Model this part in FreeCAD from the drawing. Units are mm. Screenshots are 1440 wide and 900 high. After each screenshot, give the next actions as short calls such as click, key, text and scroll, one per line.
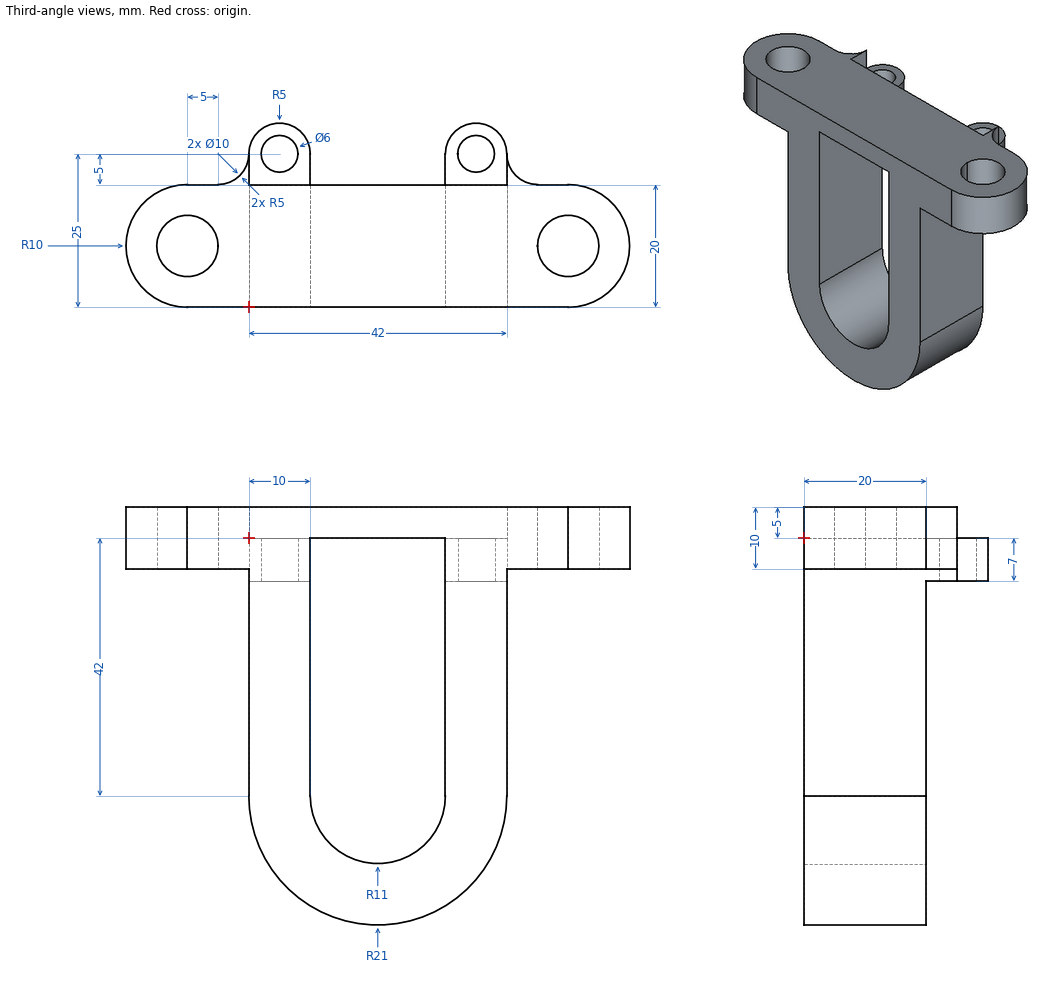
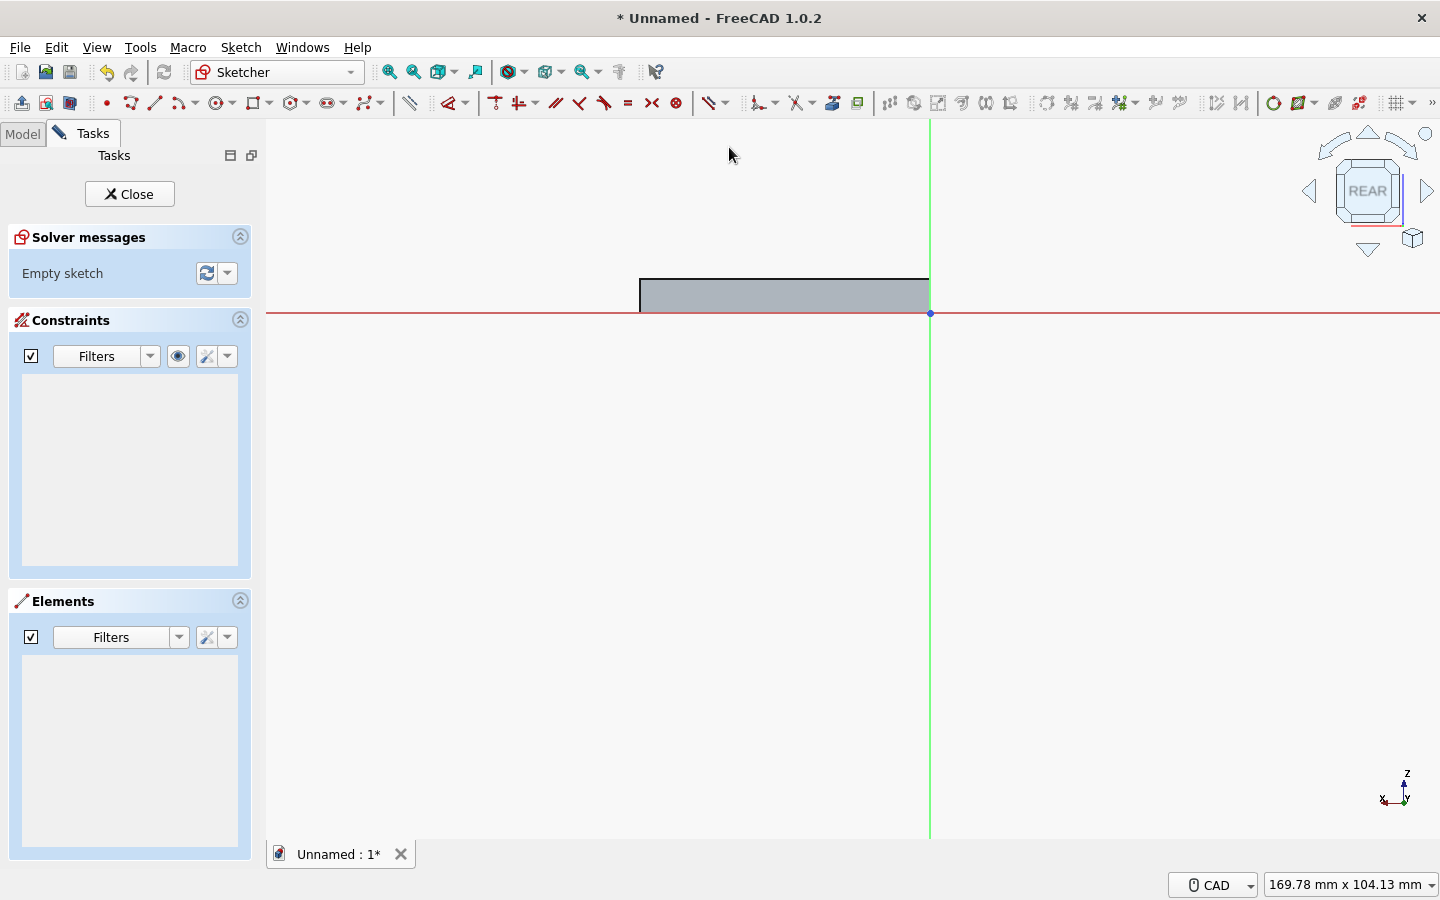
click(132, 104)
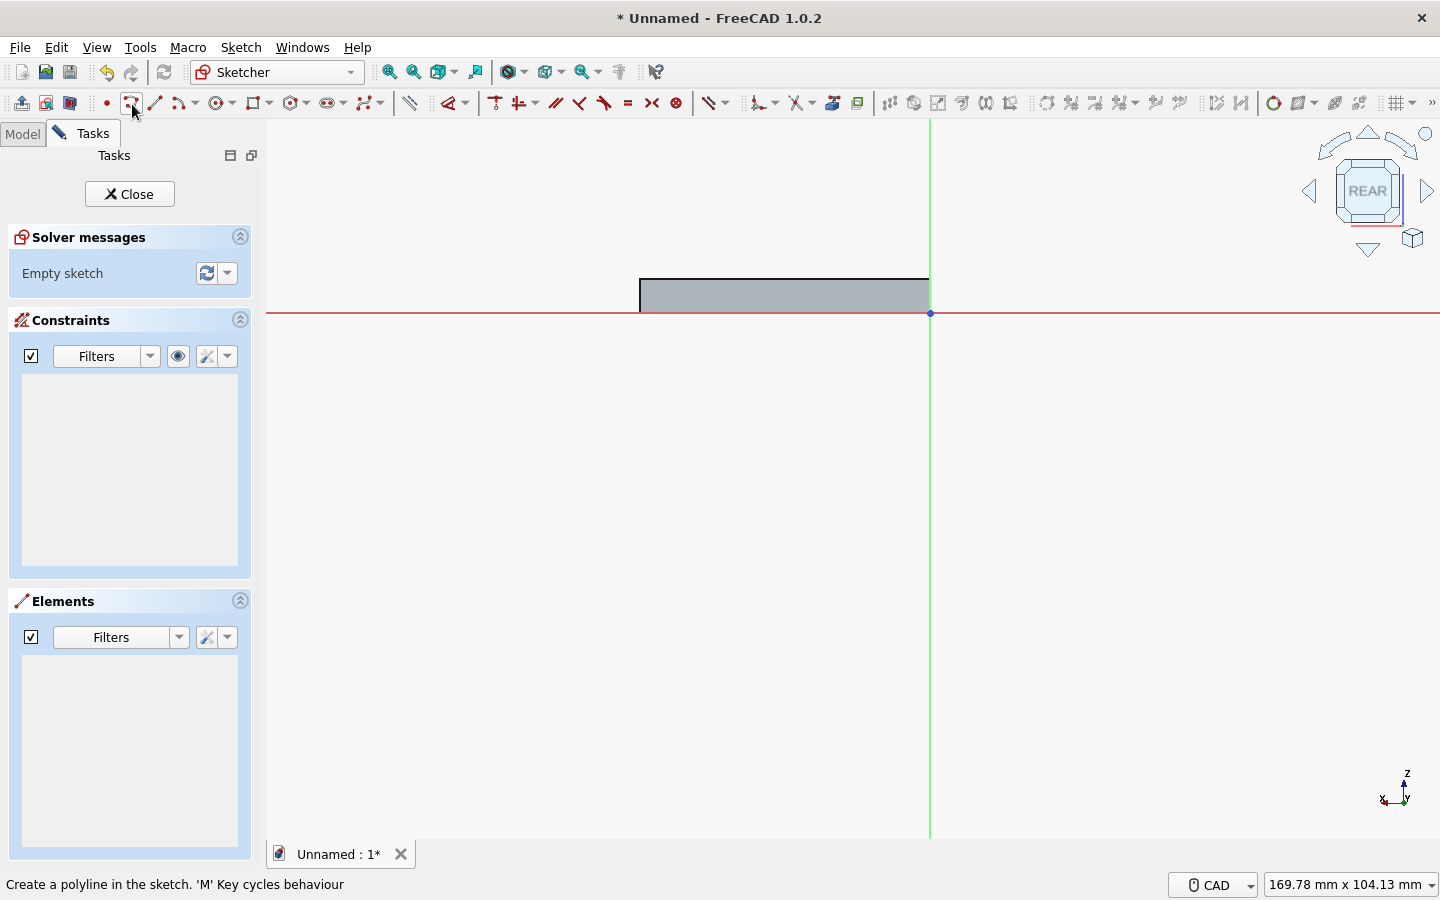
click(930, 604)
click(930, 313)
click(640, 322)
click(640, 604)
right_click(640, 604)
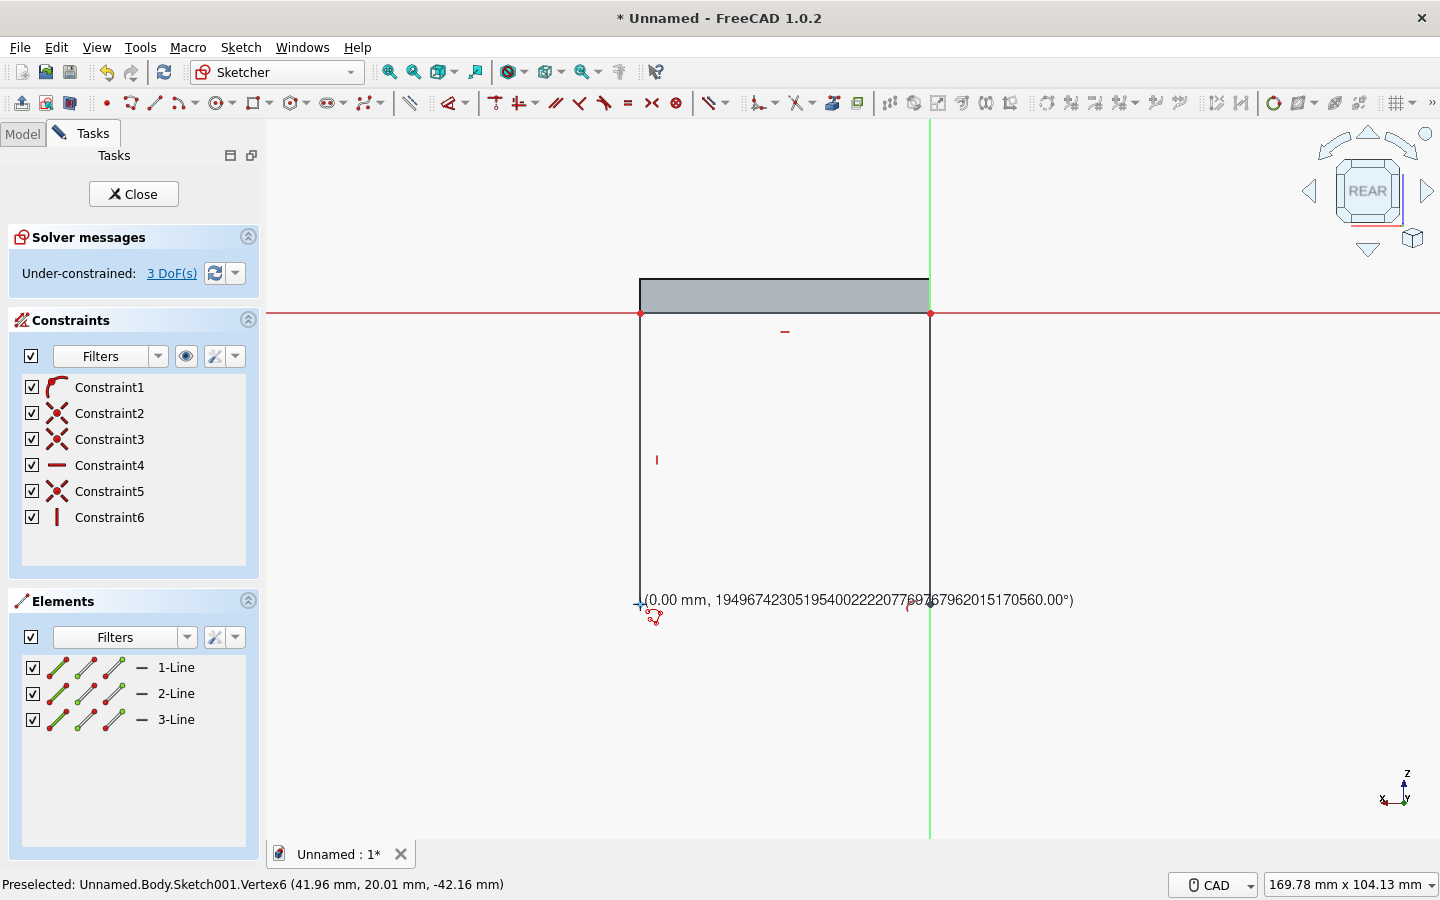
click(198, 104)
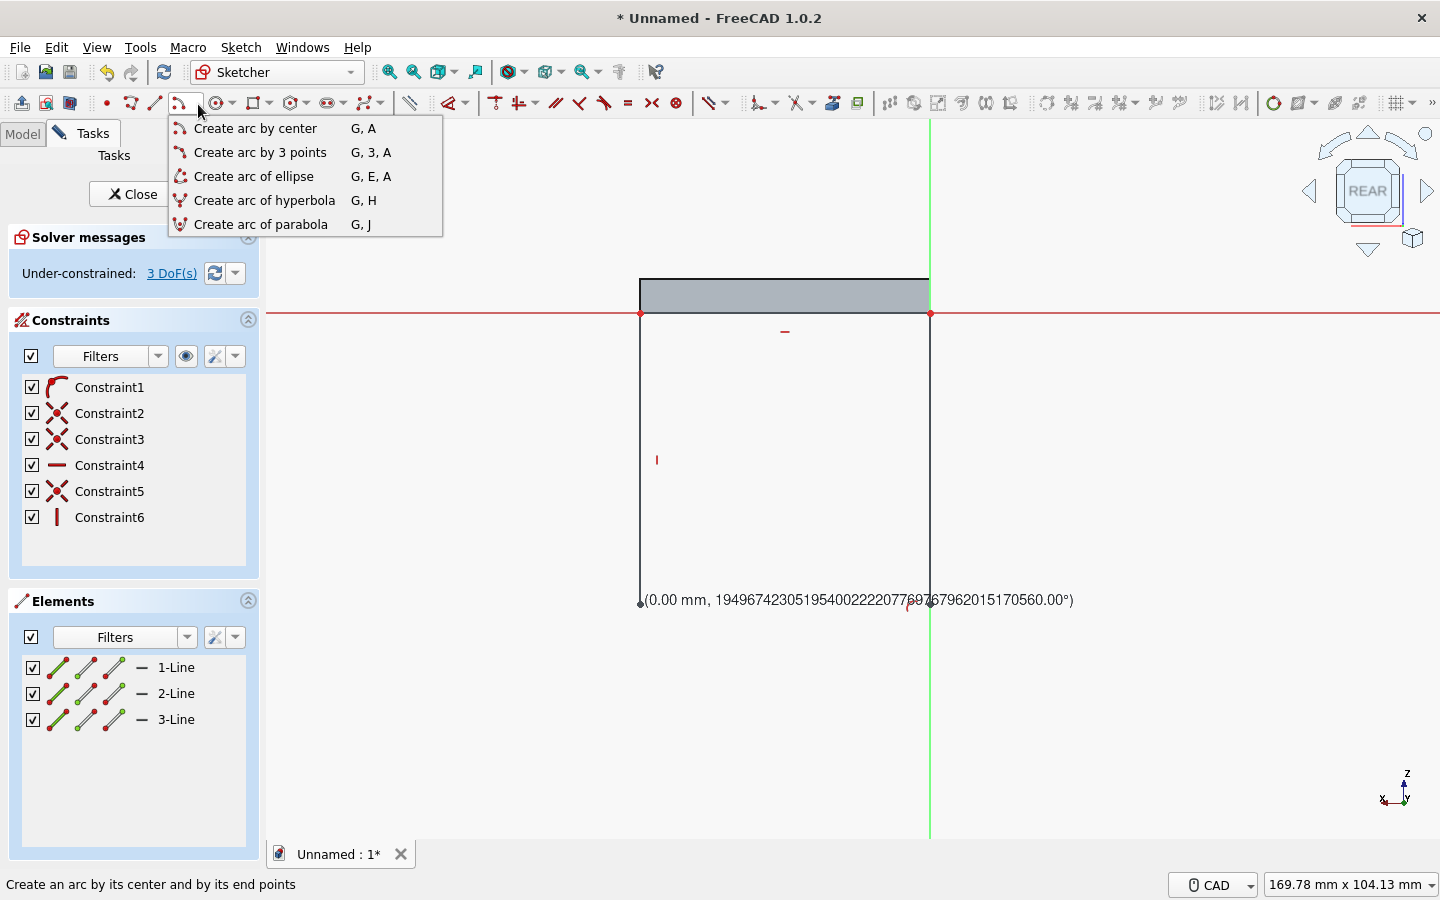
click(306, 152)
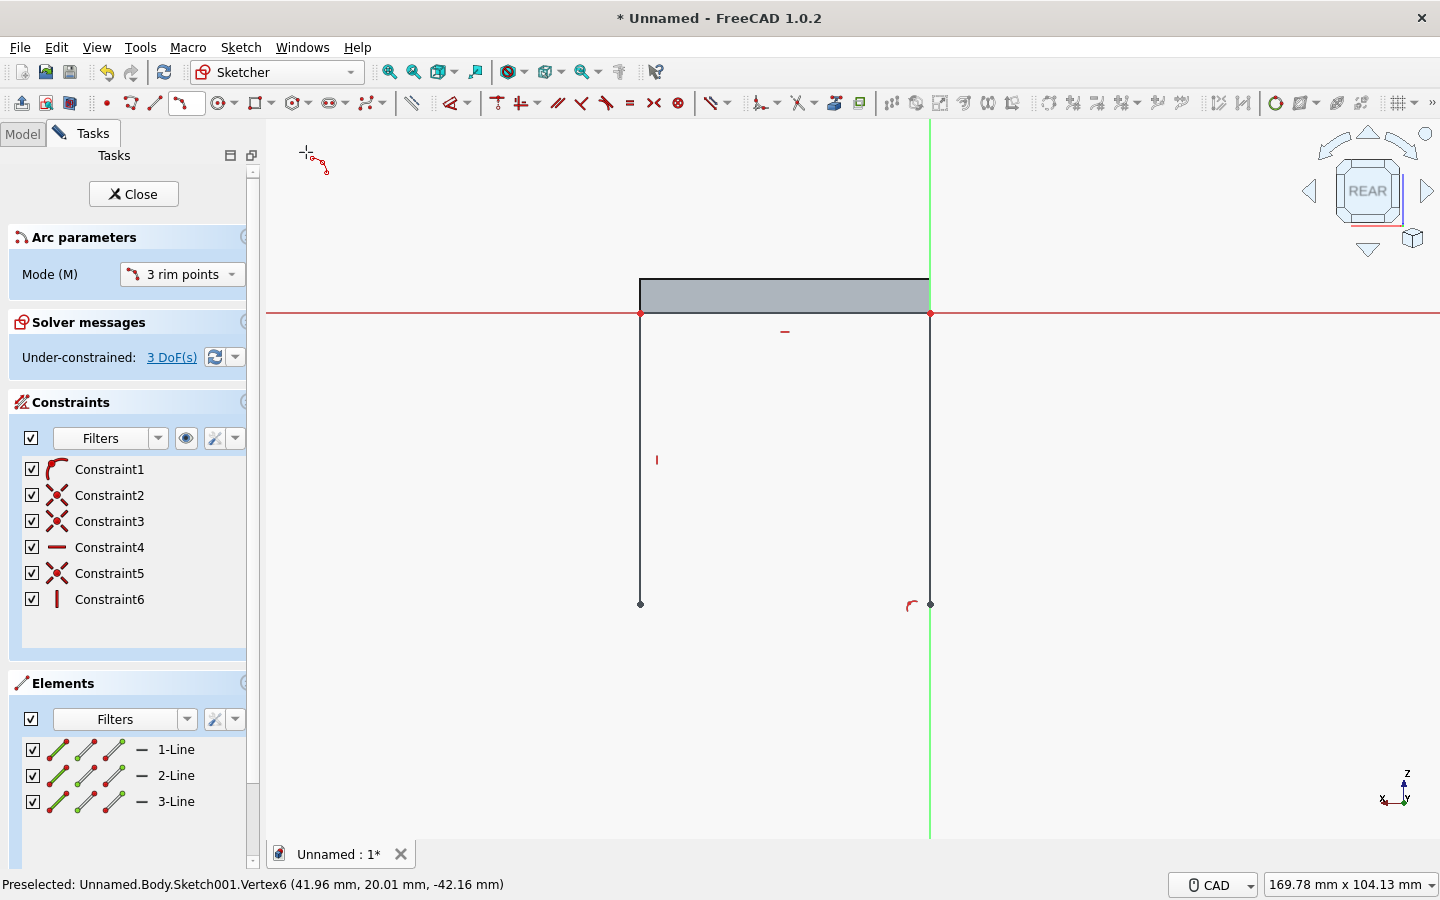
click(640, 605)
click(930, 605)
click(785, 749)
key(Escape)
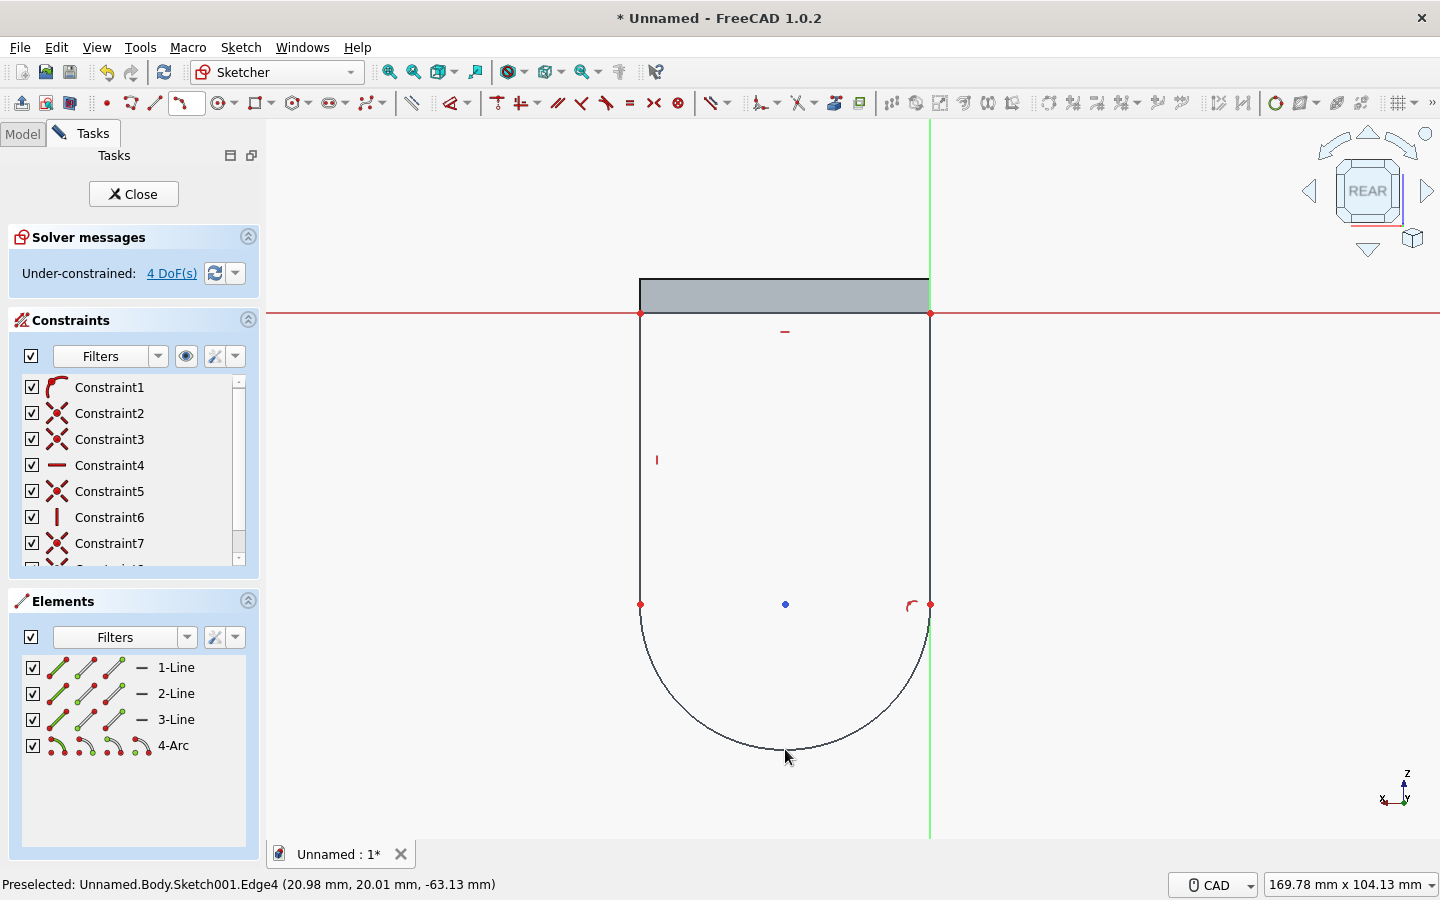
click(930, 518)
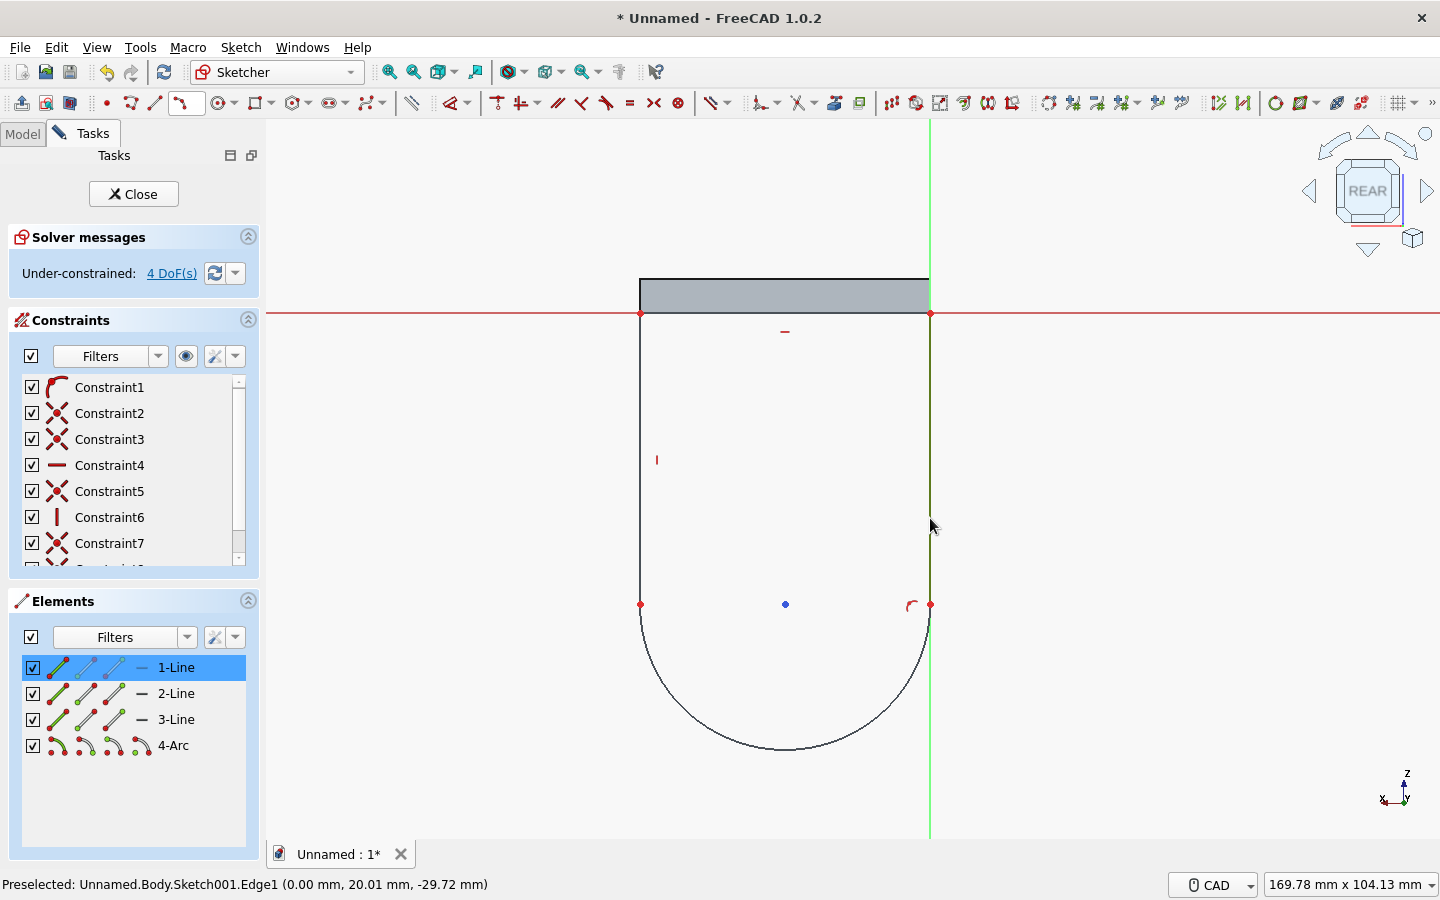
click(700, 722)